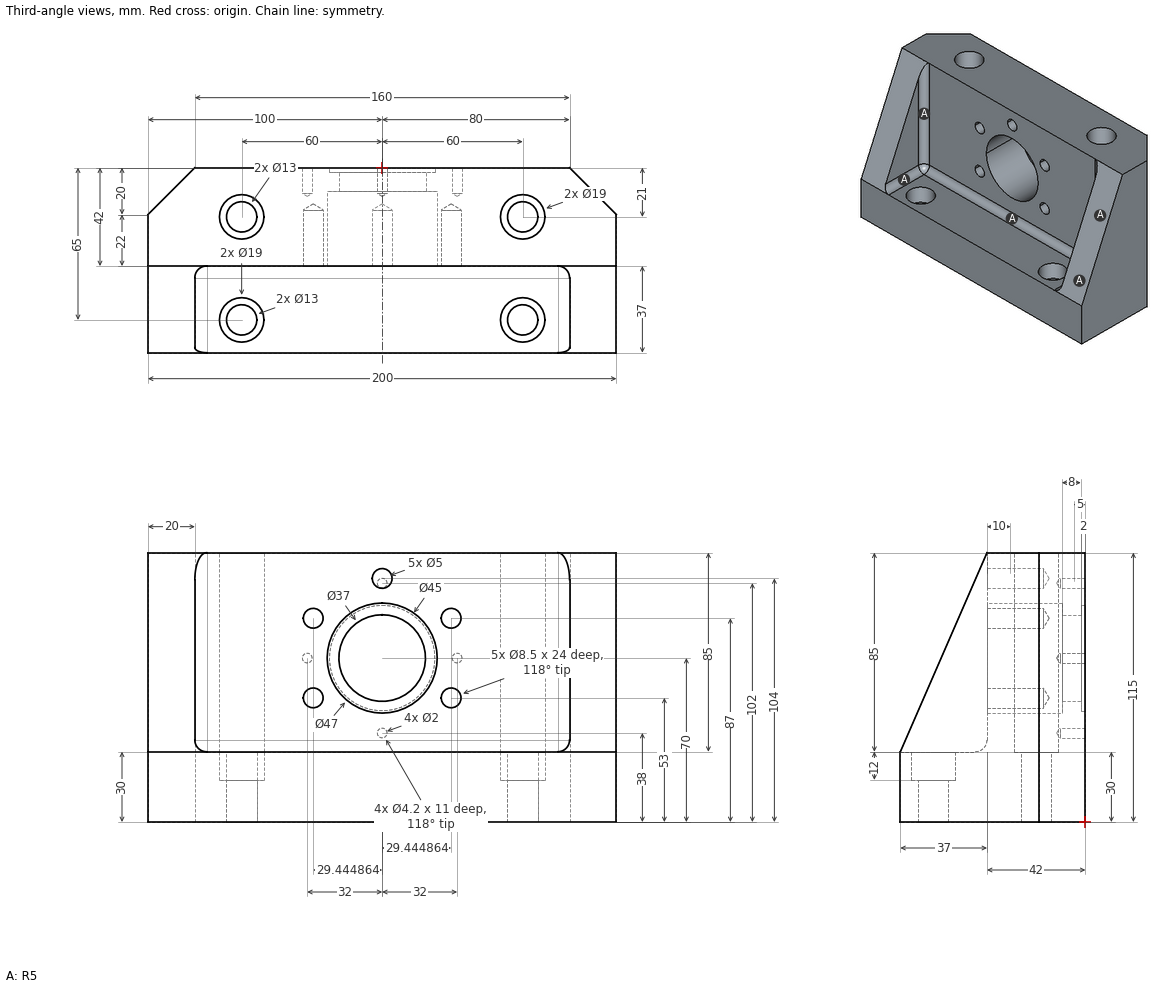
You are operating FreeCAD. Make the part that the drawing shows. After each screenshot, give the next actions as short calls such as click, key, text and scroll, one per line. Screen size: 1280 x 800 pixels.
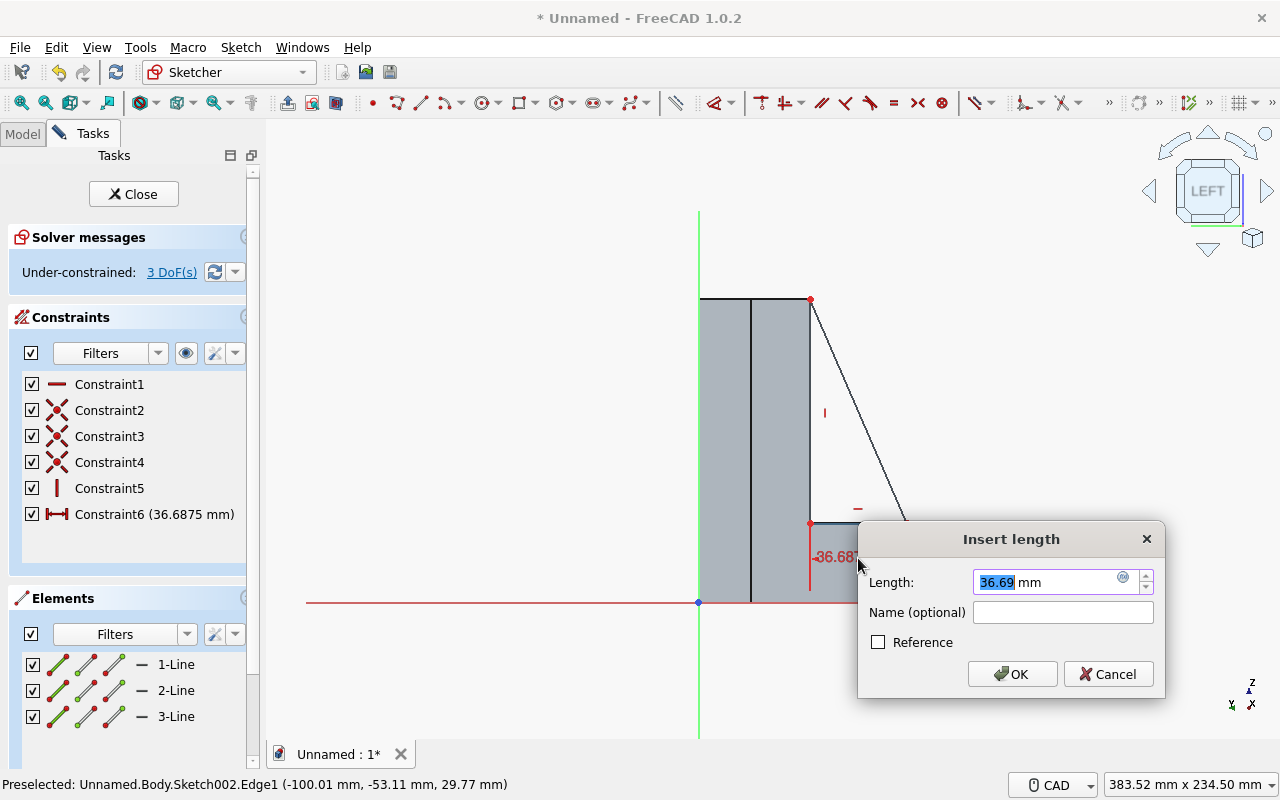
text(37)
key(Return)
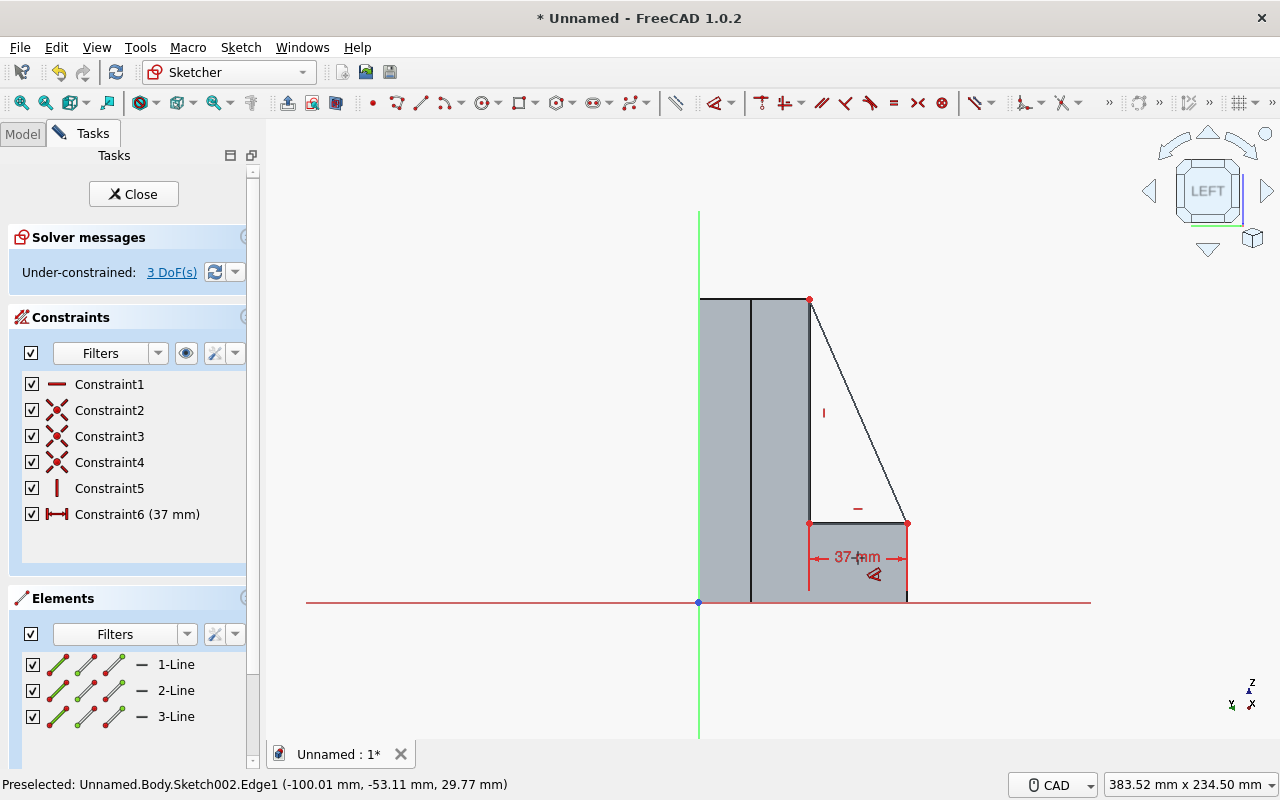
click(809, 367)
click(843, 412)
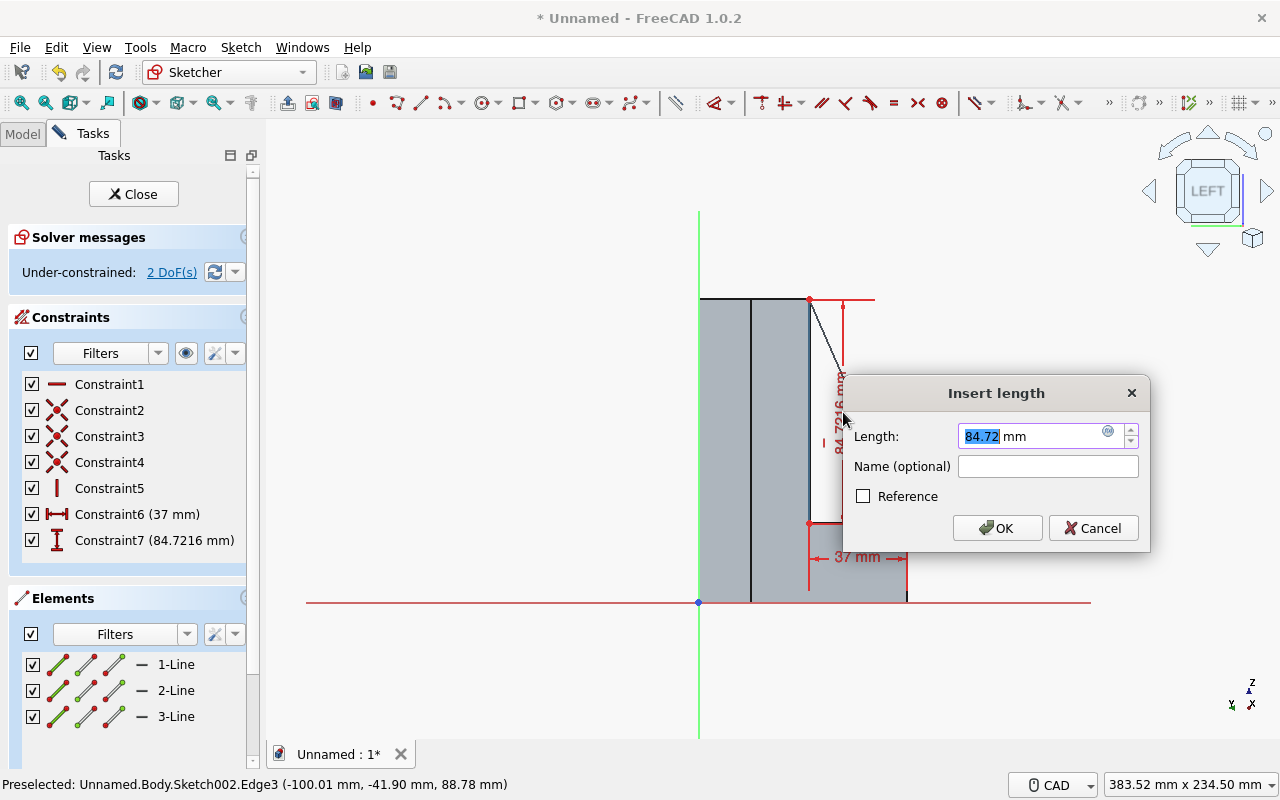
text(85)
key(Return)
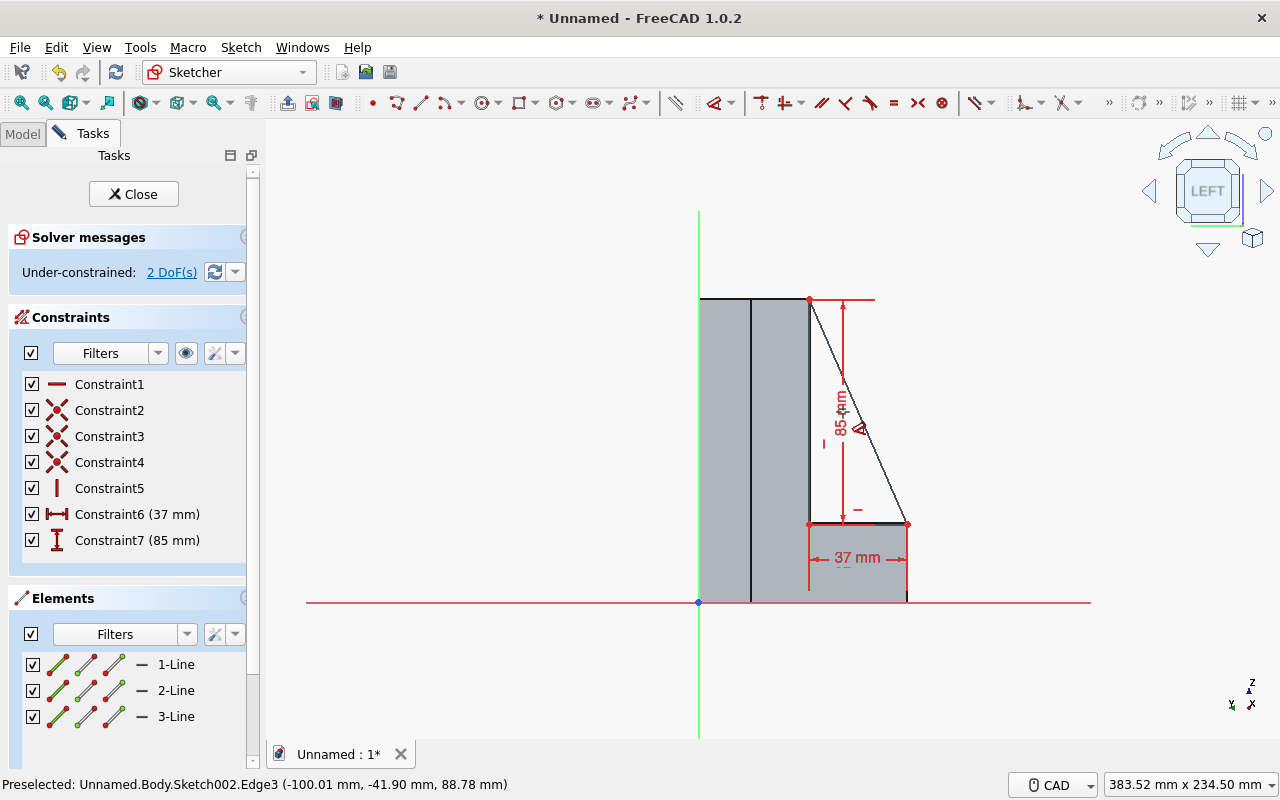
click(809, 525)
click(754, 637)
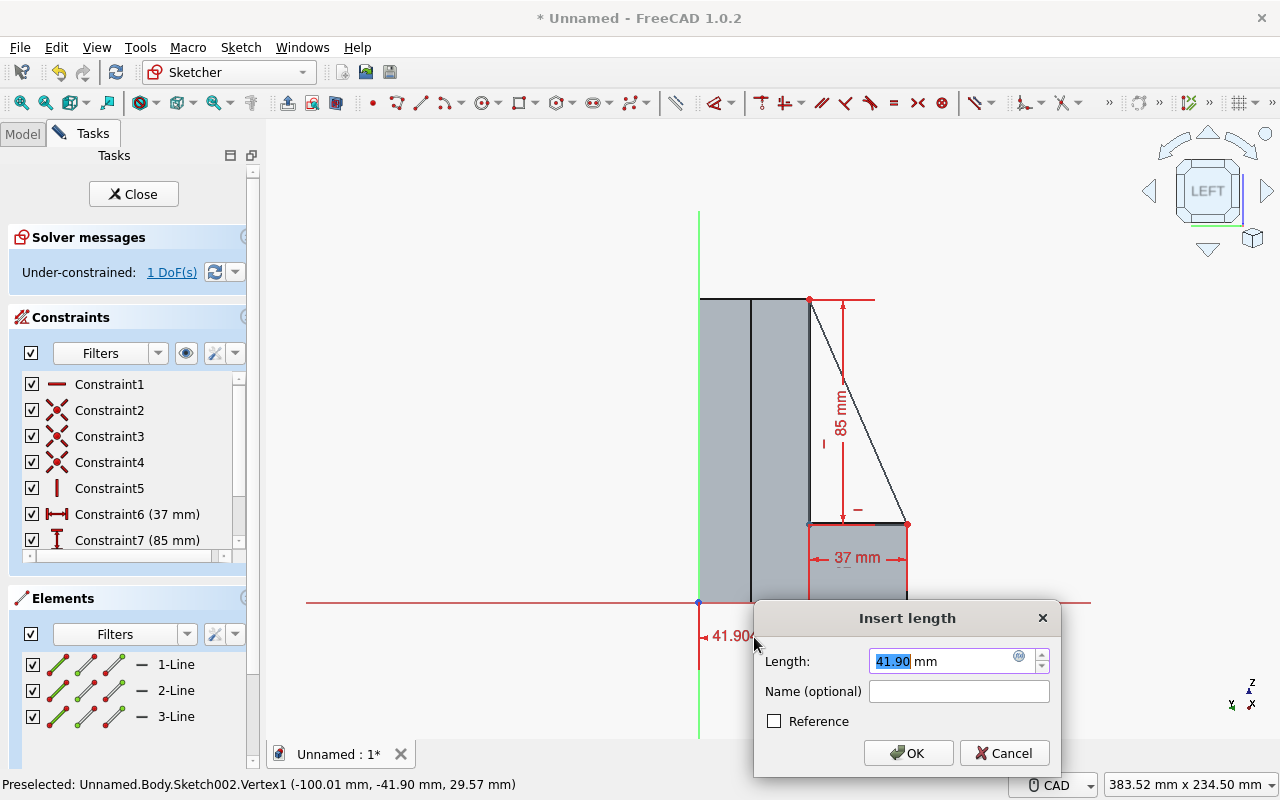
text(42)
key(Return)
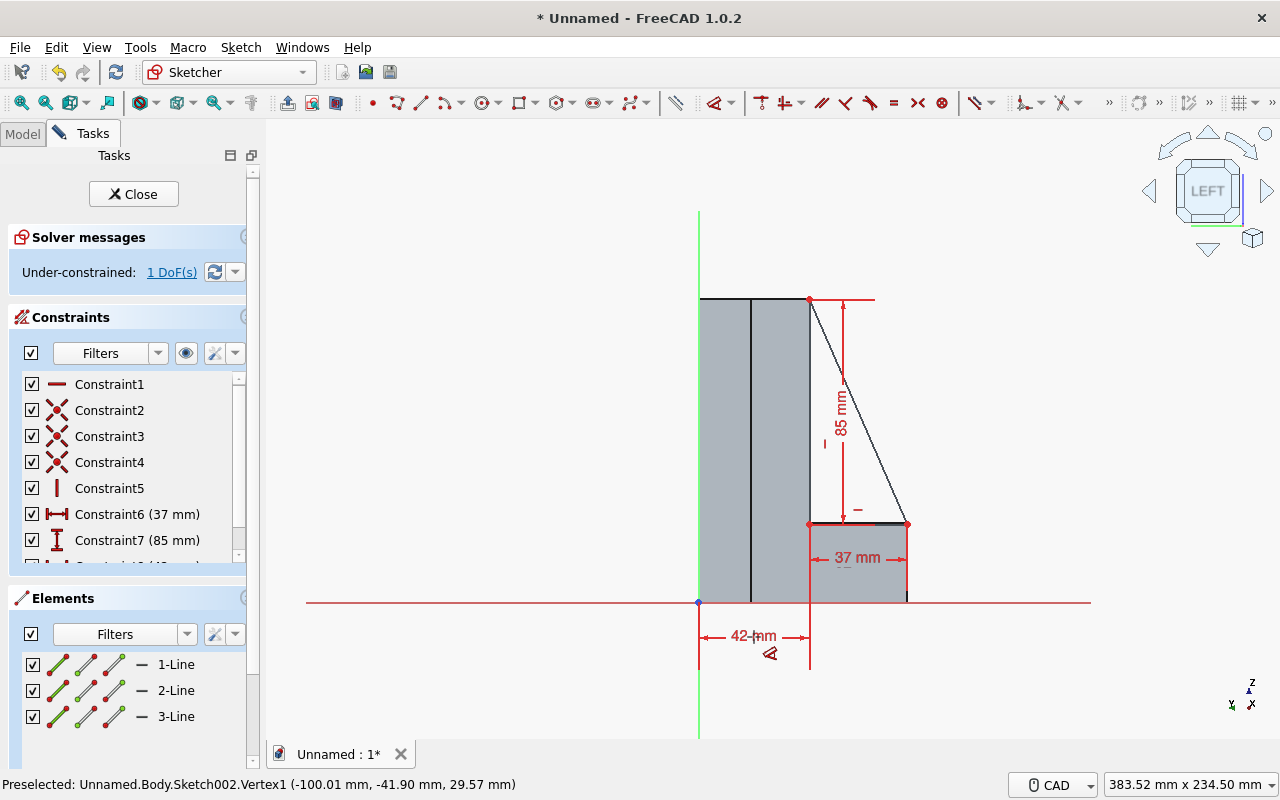
click(810, 525)
click(665, 564)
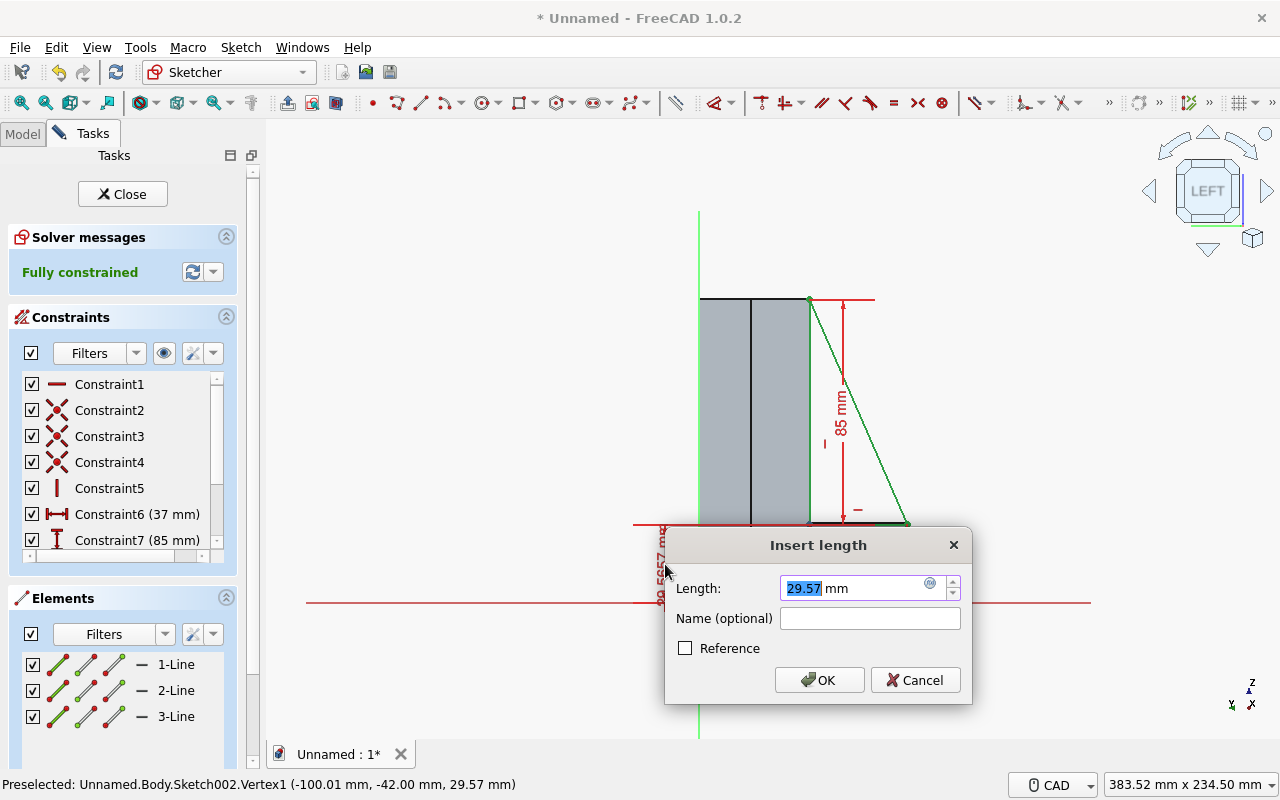
text(30)
key(Return)
key(Escape)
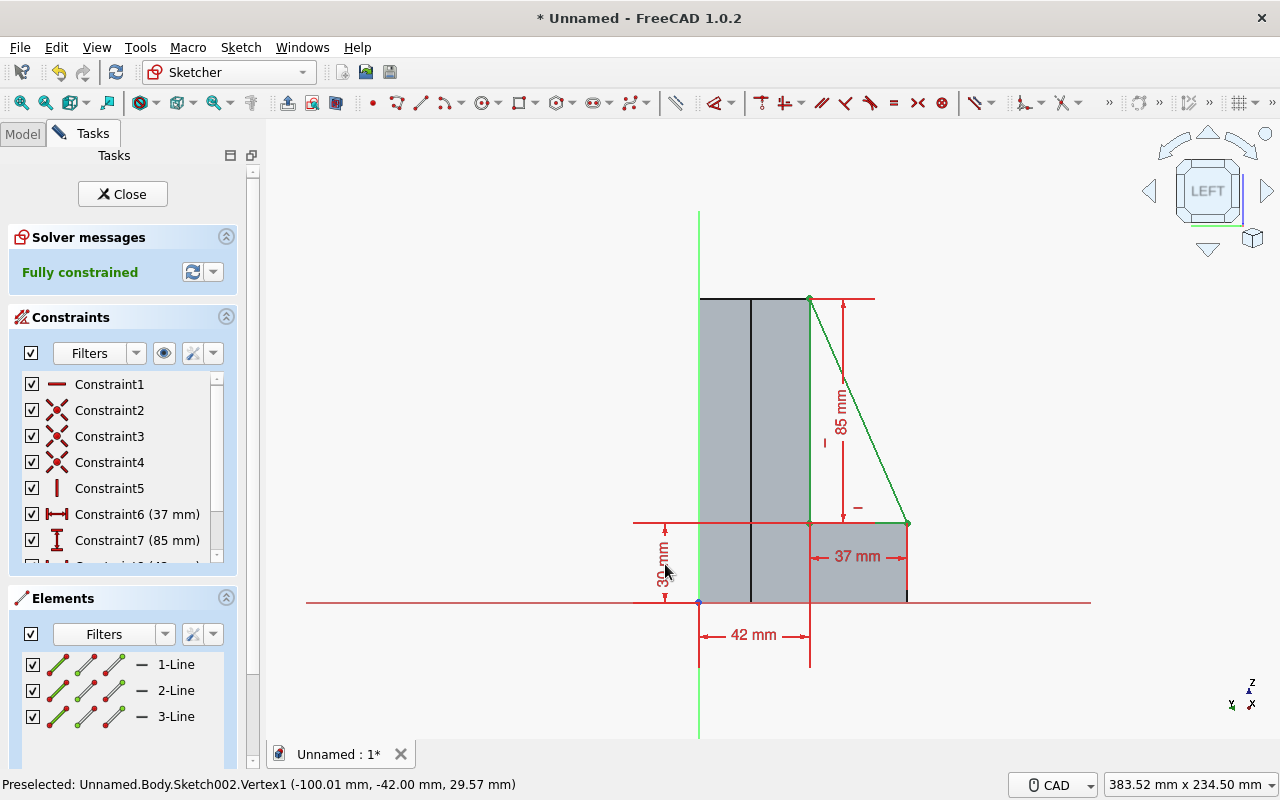
click(123, 194)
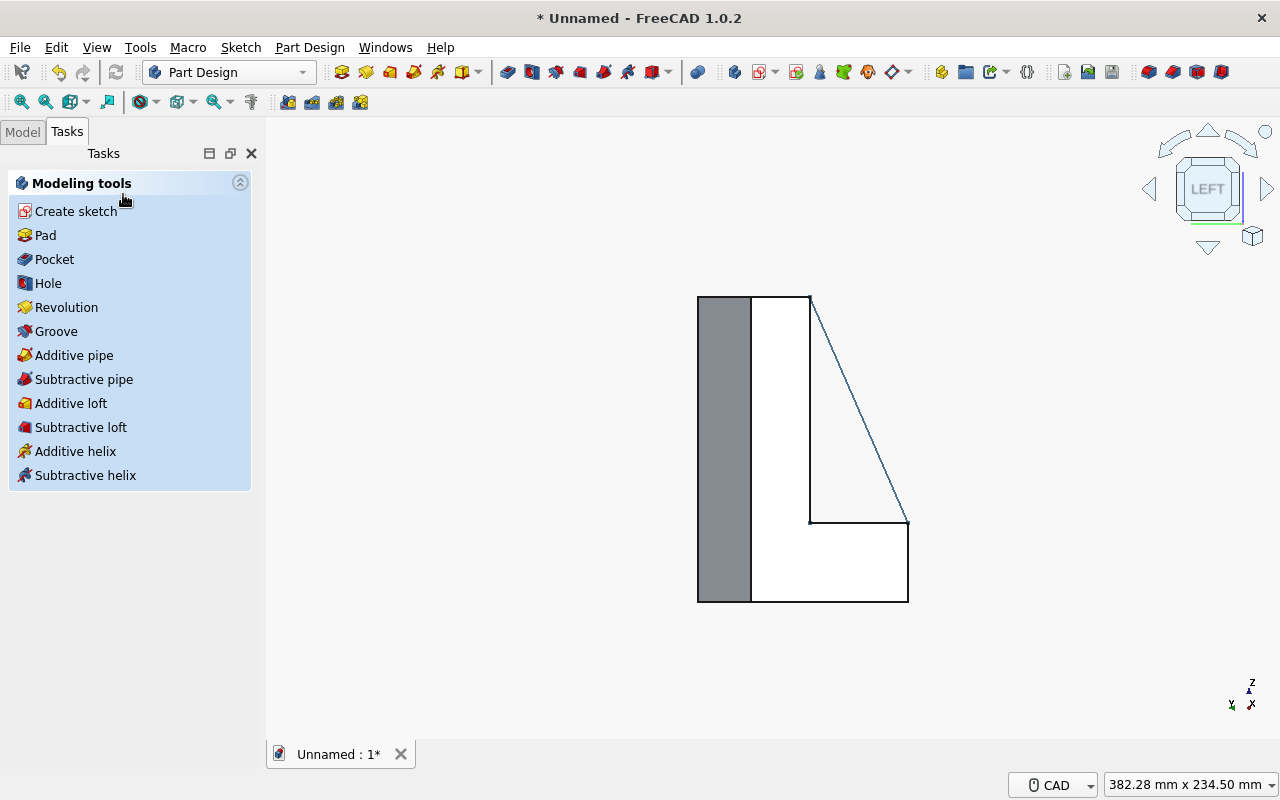
click(342, 72)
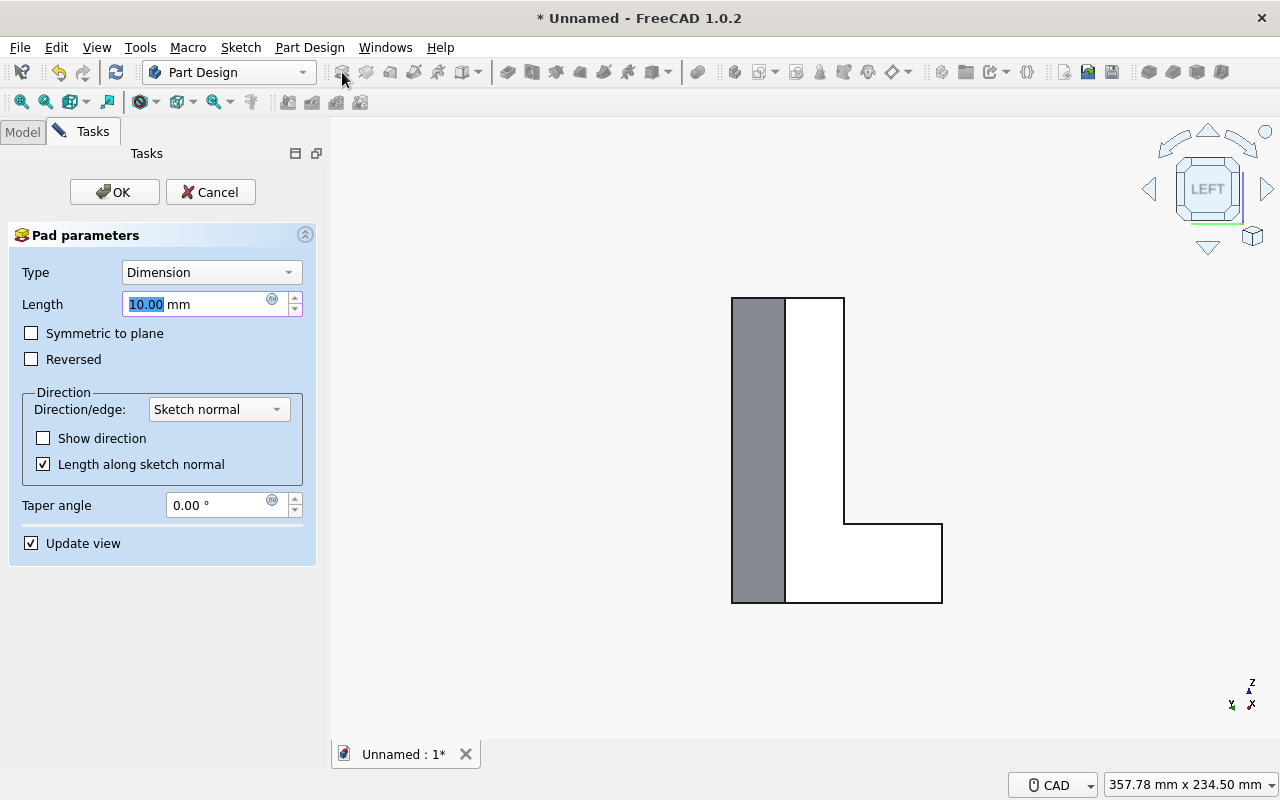
text(20)
key(Tab)